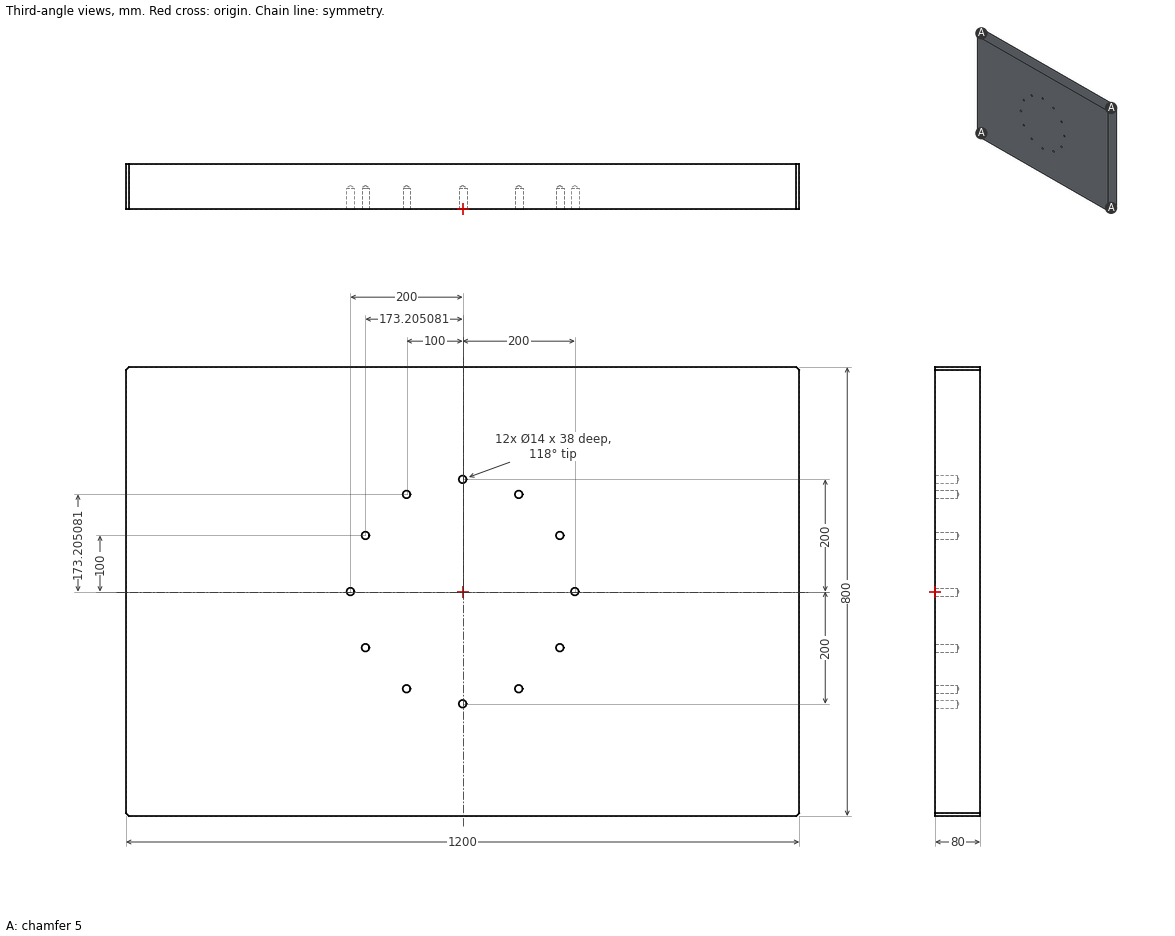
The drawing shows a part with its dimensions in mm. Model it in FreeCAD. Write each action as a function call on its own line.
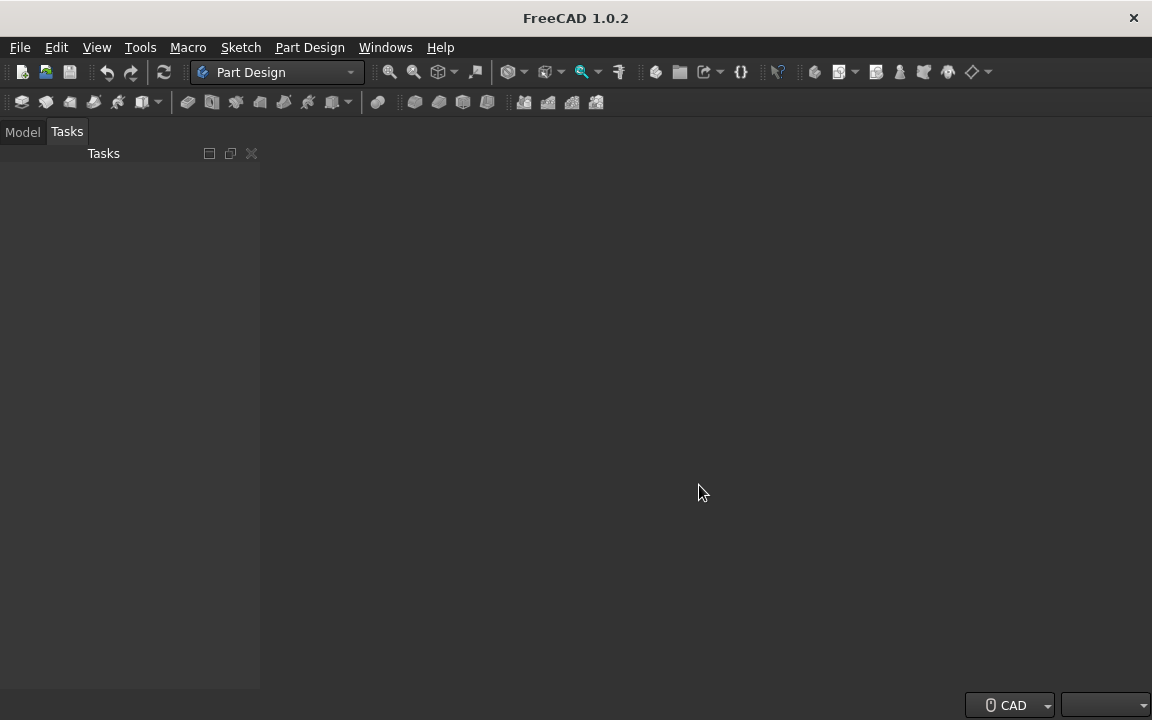
click(22, 72)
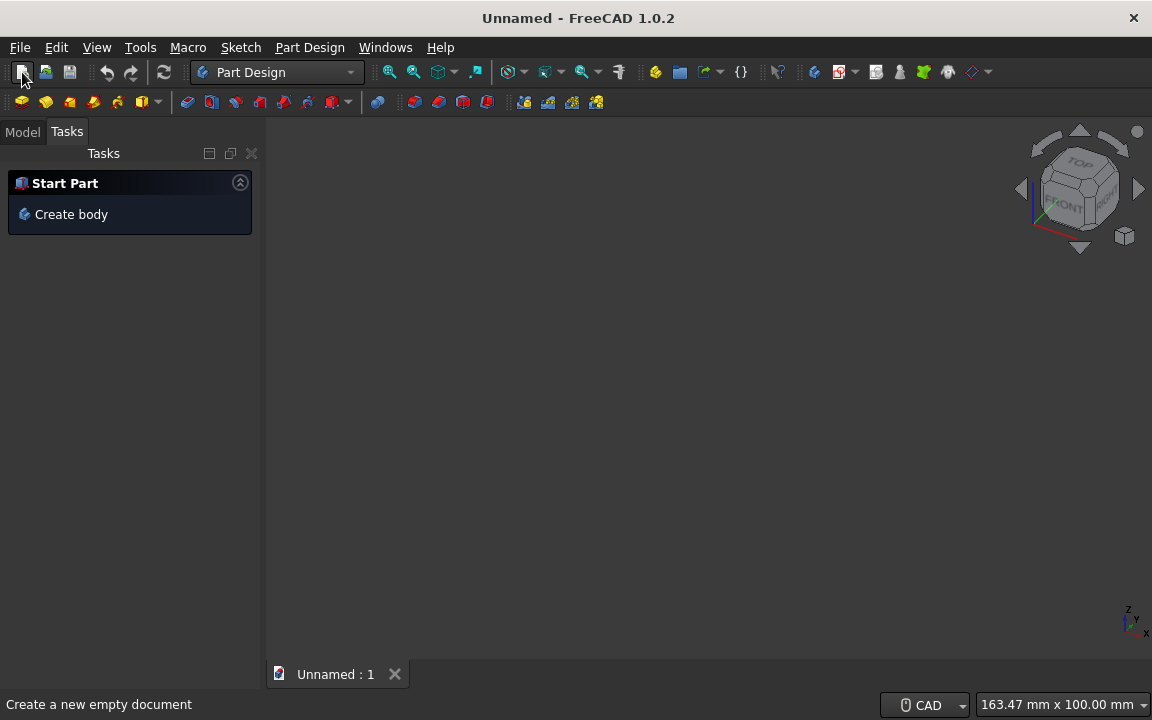
click(840, 72)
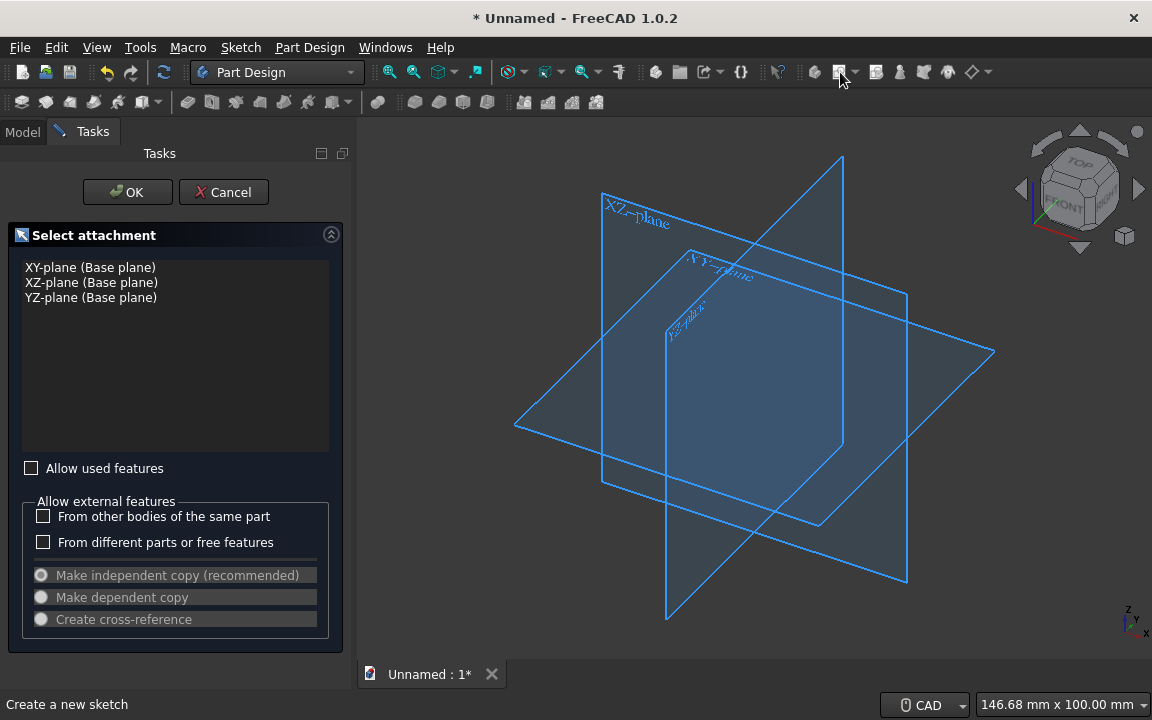
click(82, 282)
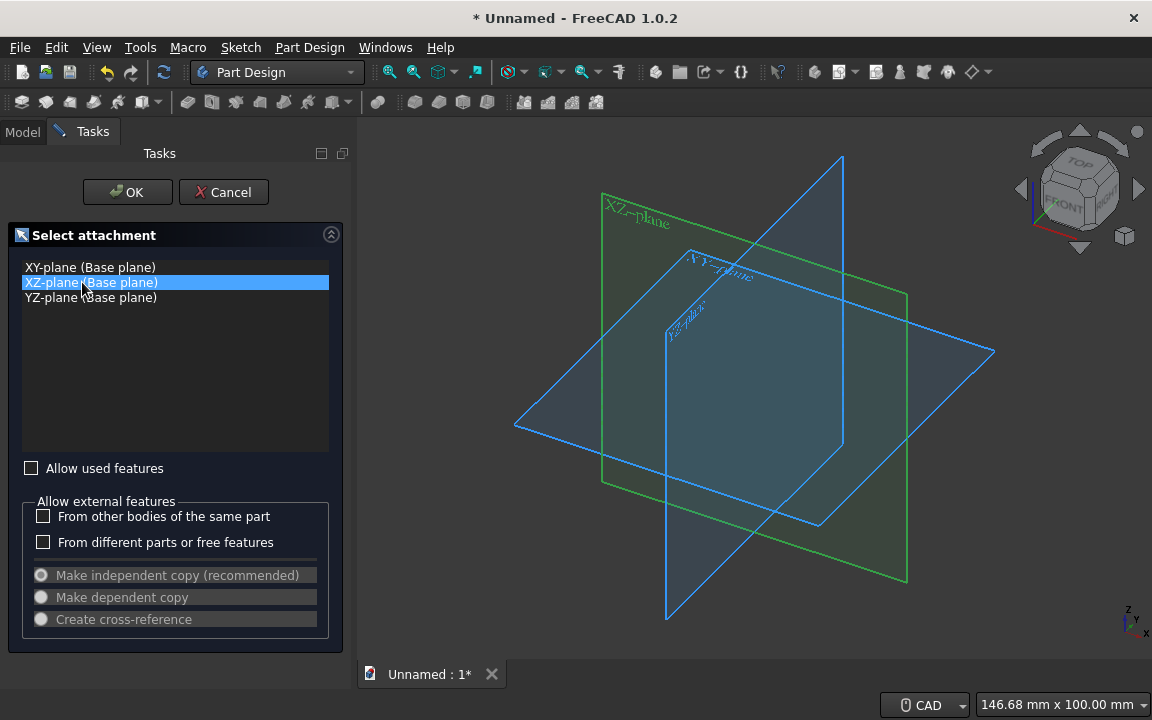
click(128, 192)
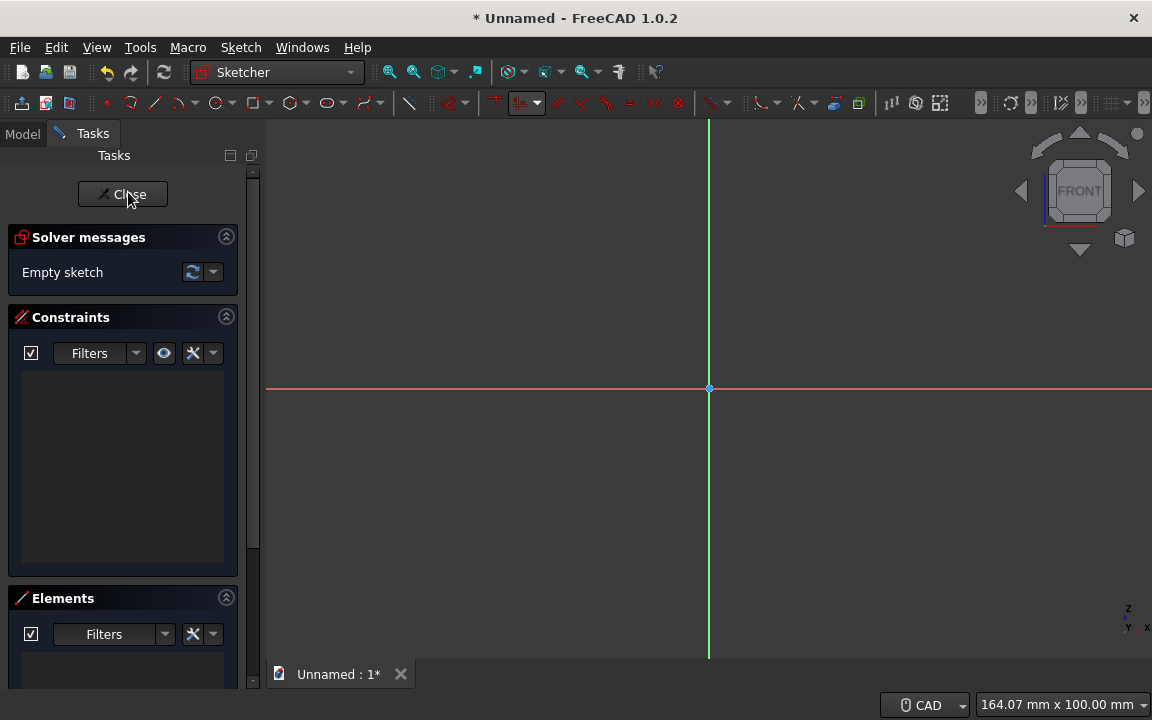
scroll(635, 389, down, 13)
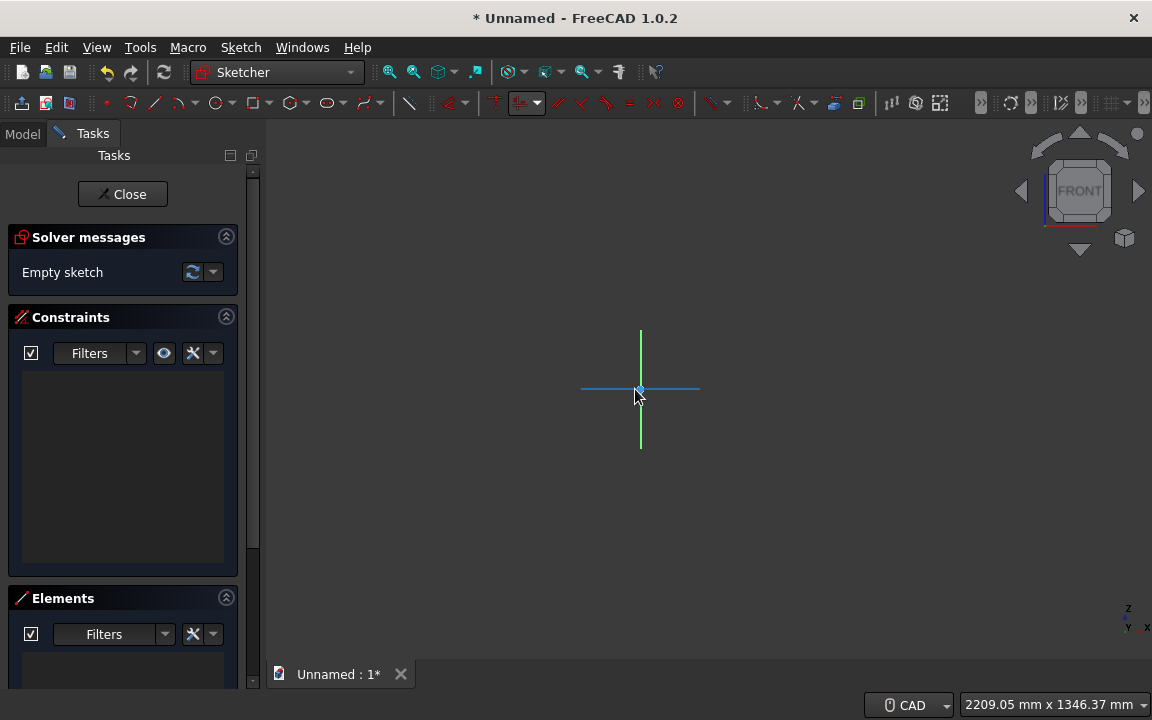
click(272, 104)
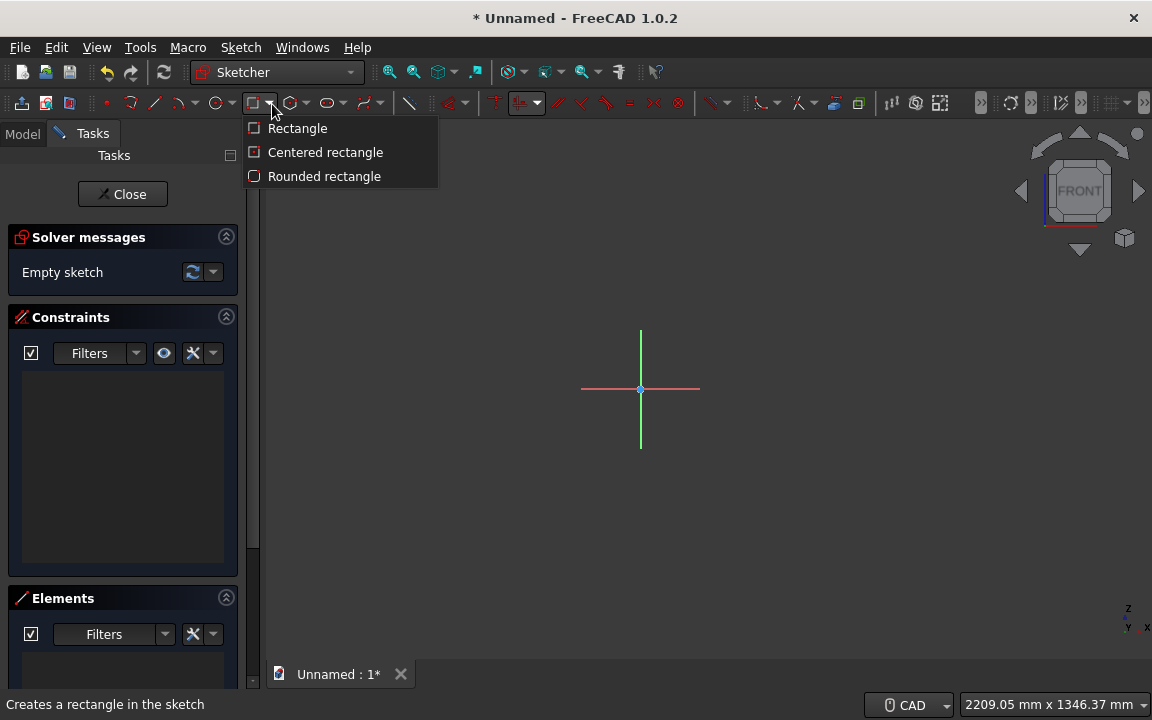
click(340, 152)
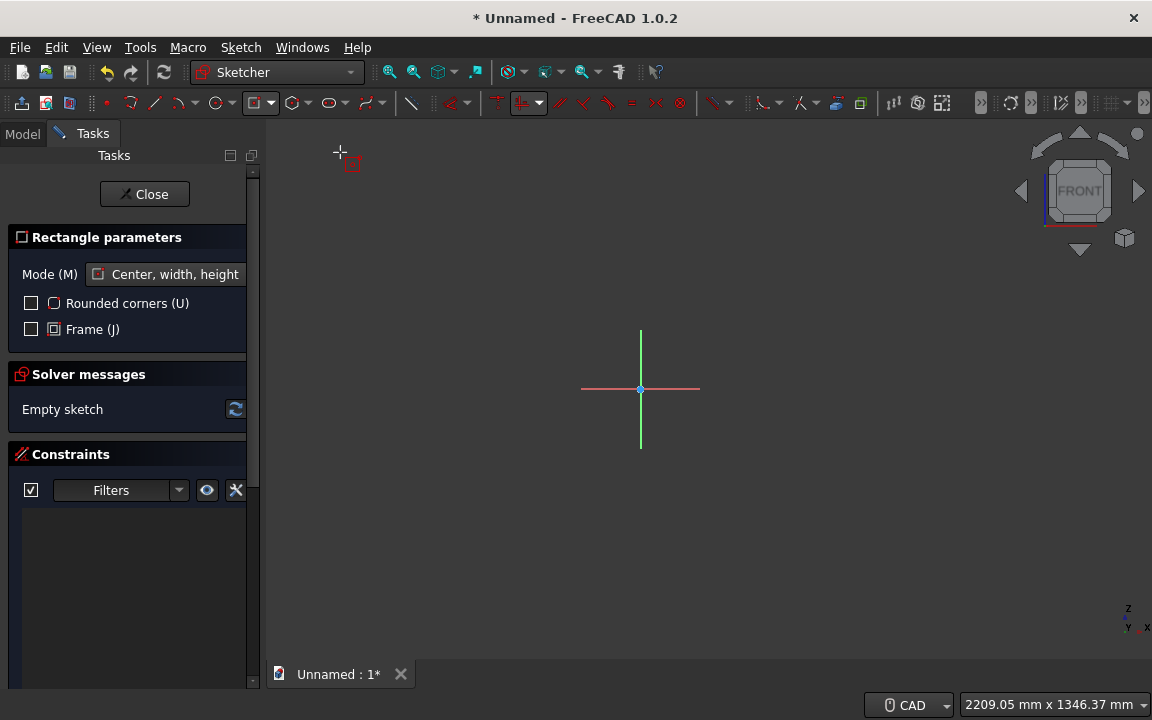
click(641, 389)
move(882, 229)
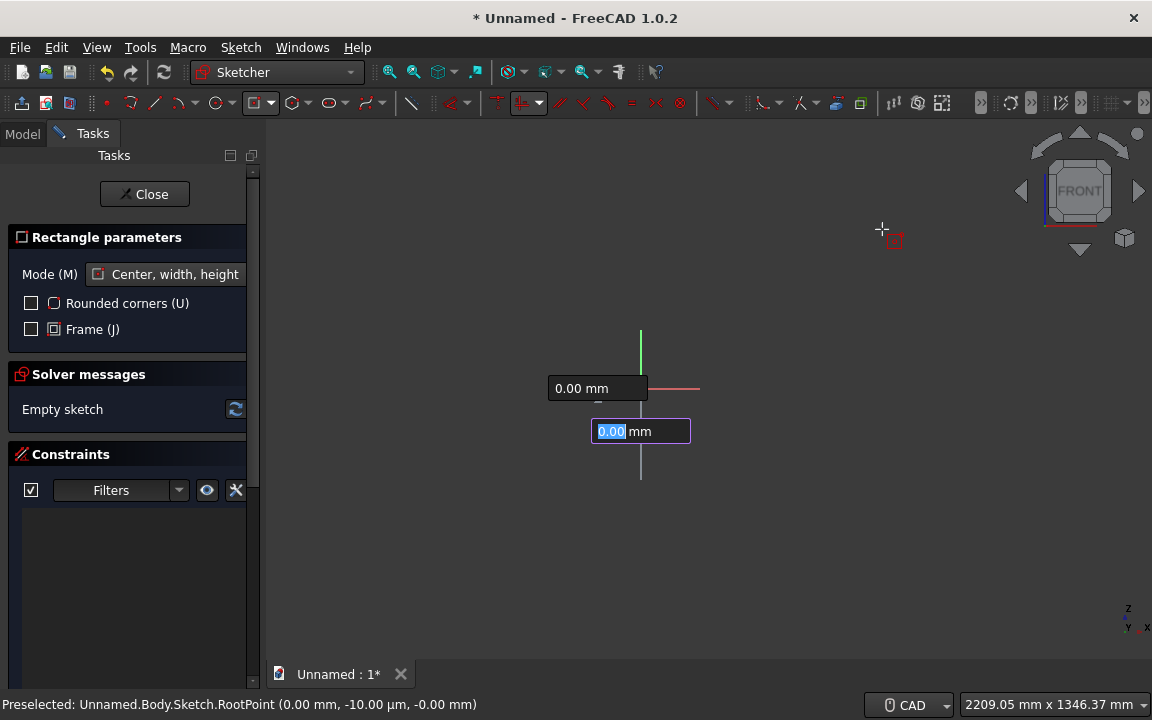
text(1200)
key(Tab)
text(800)
key(Return)
key(Escape)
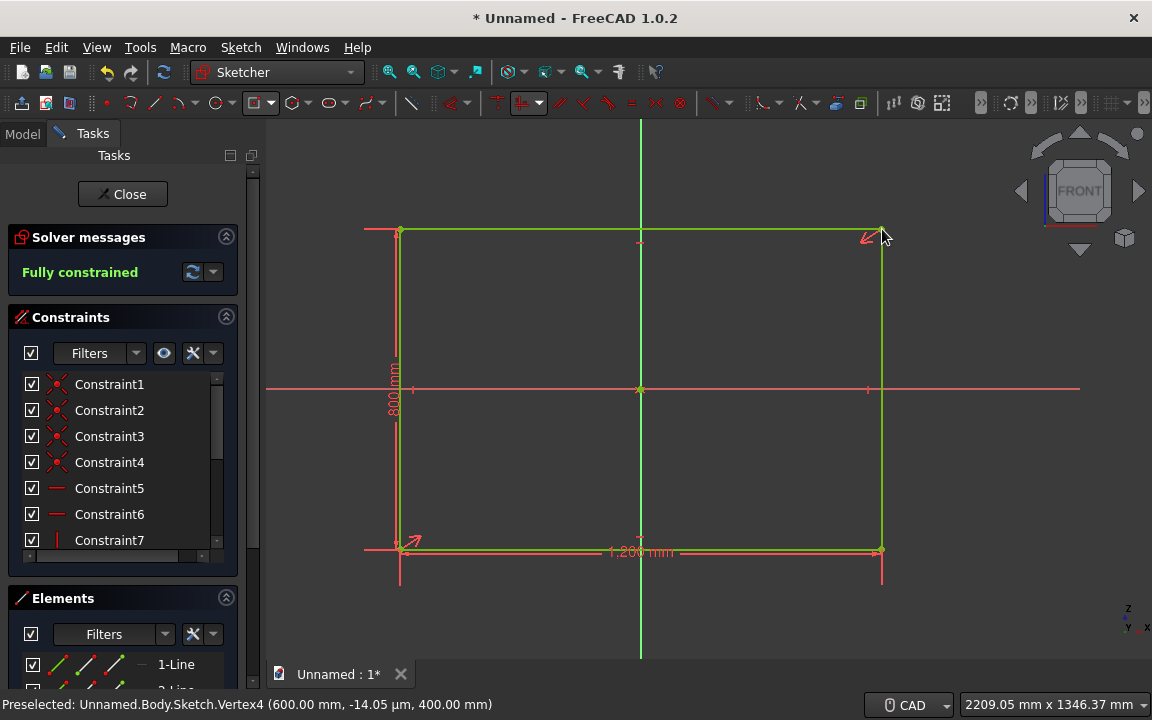
click(123, 194)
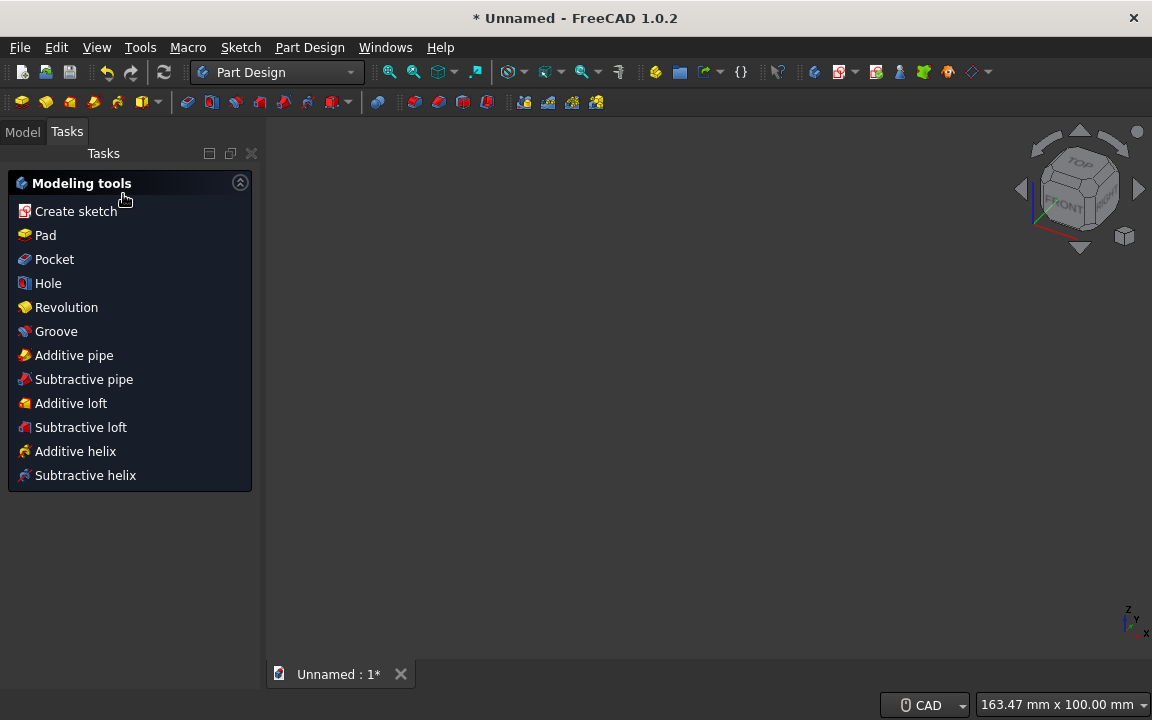
click(22, 102)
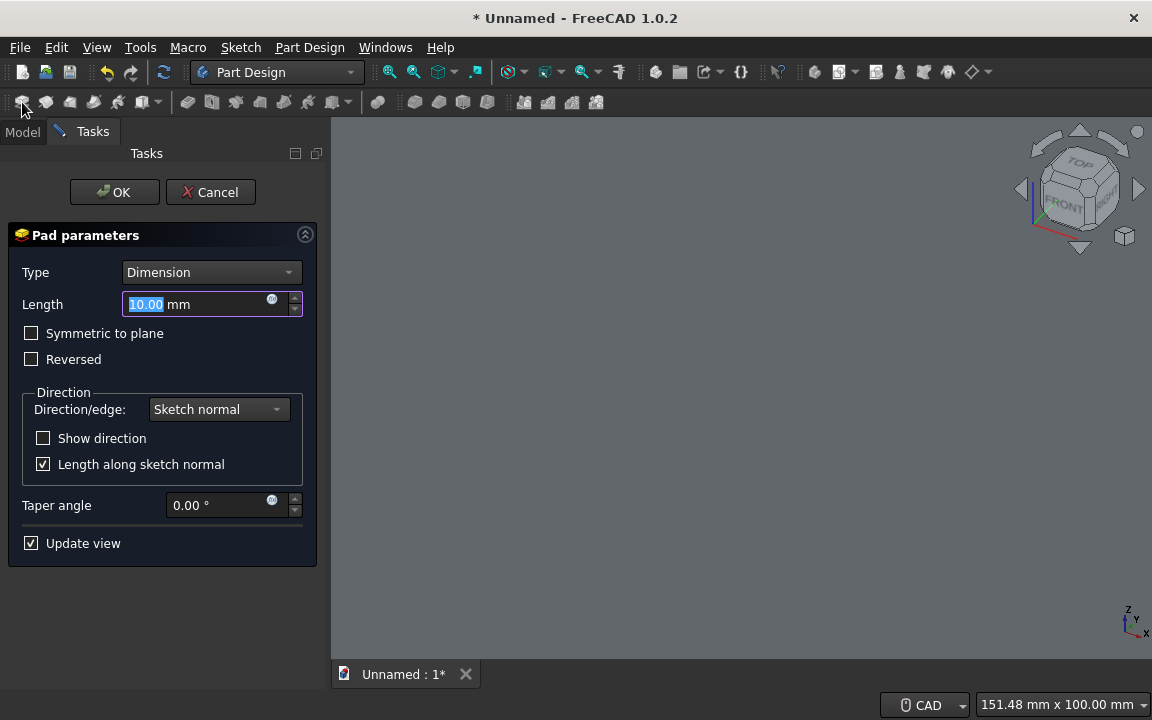
text(80)
key(Tab)